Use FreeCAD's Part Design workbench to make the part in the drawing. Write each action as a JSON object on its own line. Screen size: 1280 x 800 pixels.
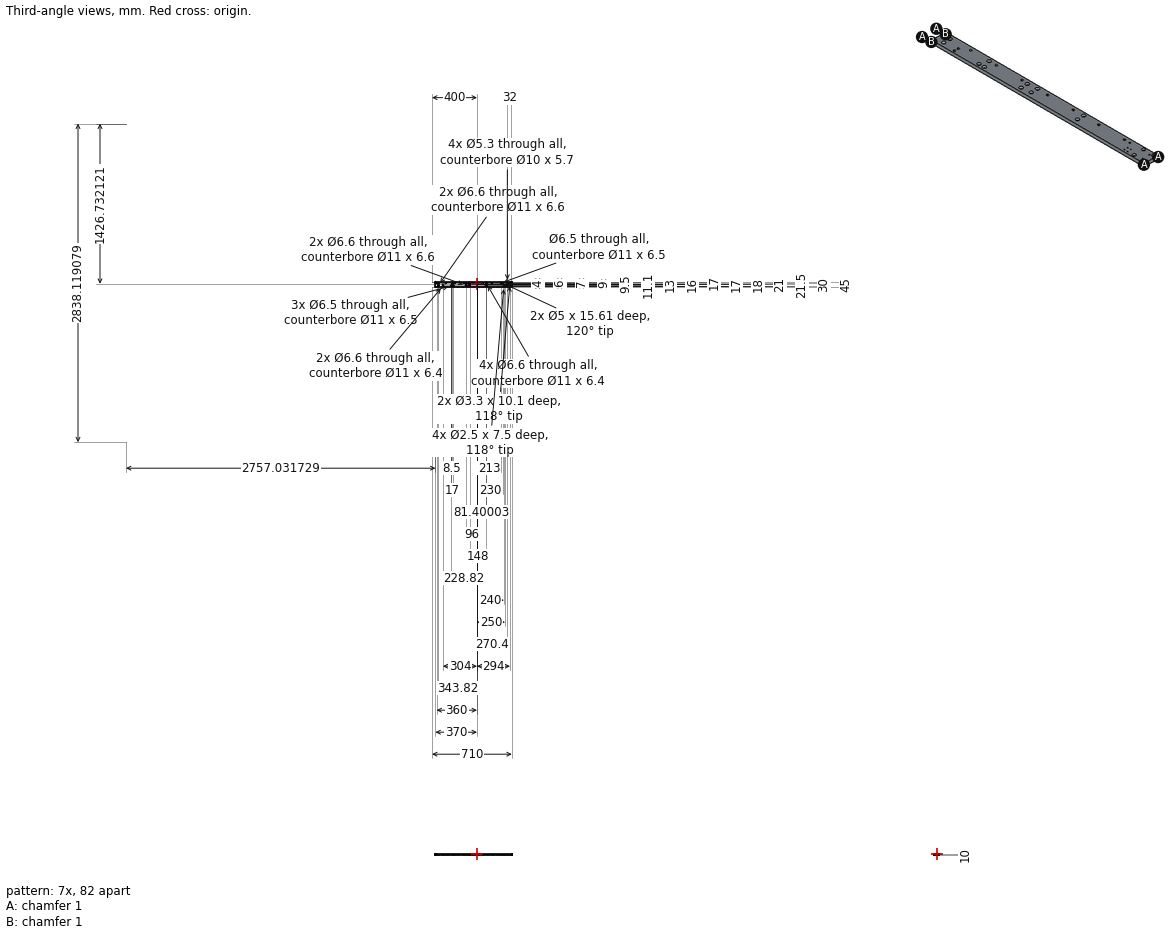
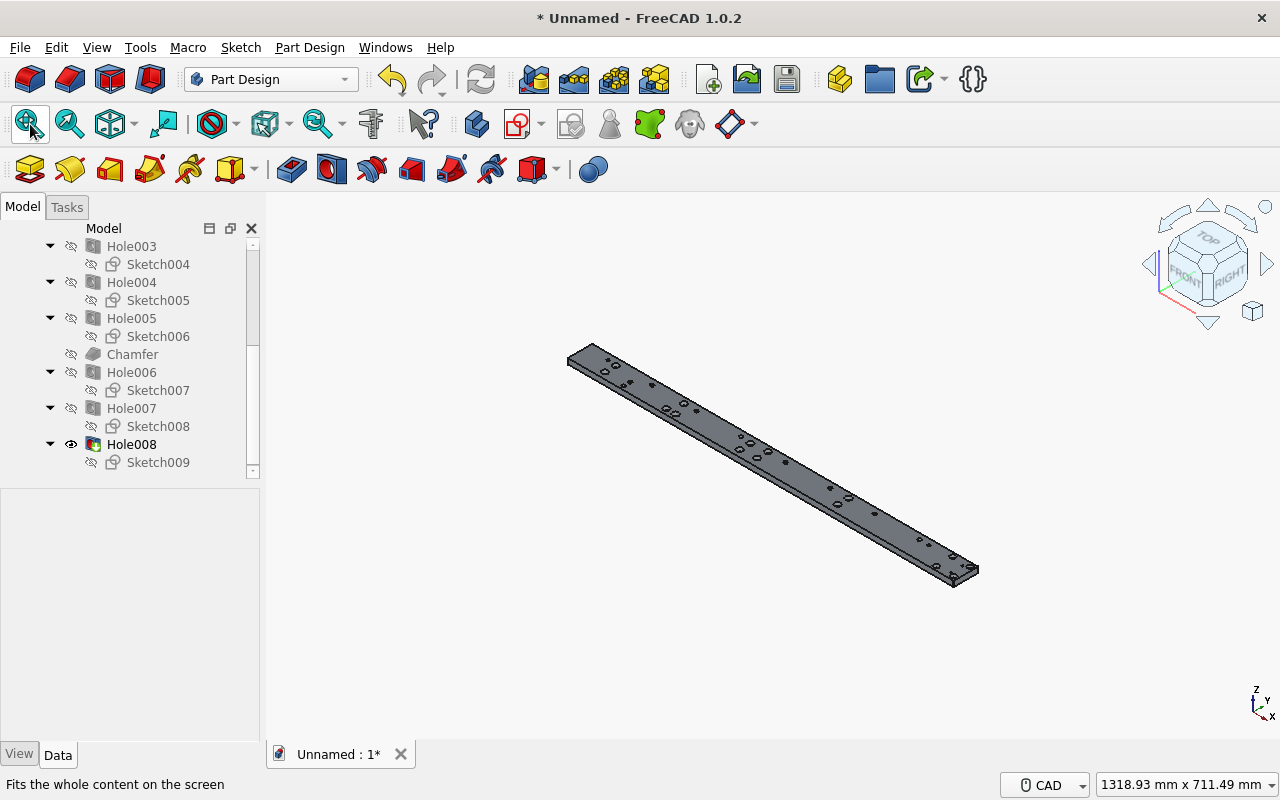
{"action": "left_click", "coordinate": [883, 525]}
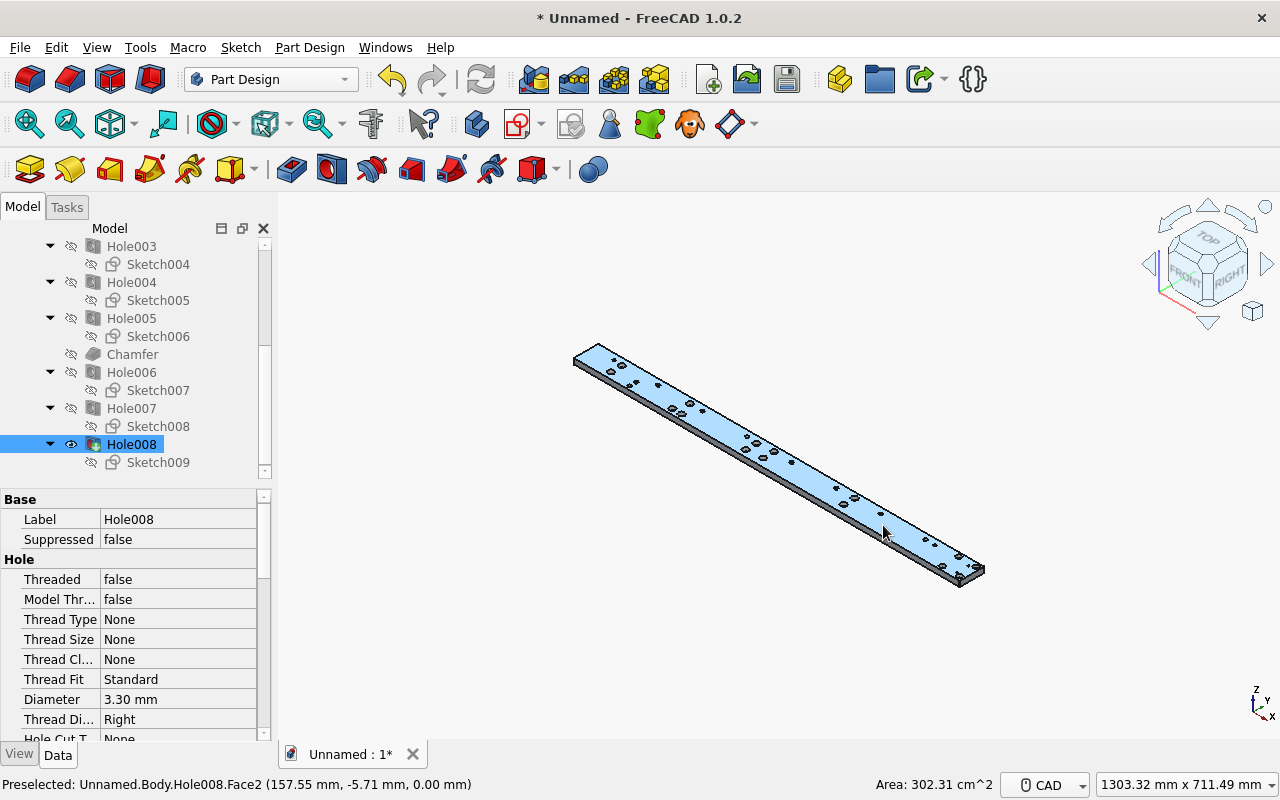
{"action": "left_click", "coordinate": [518, 124]}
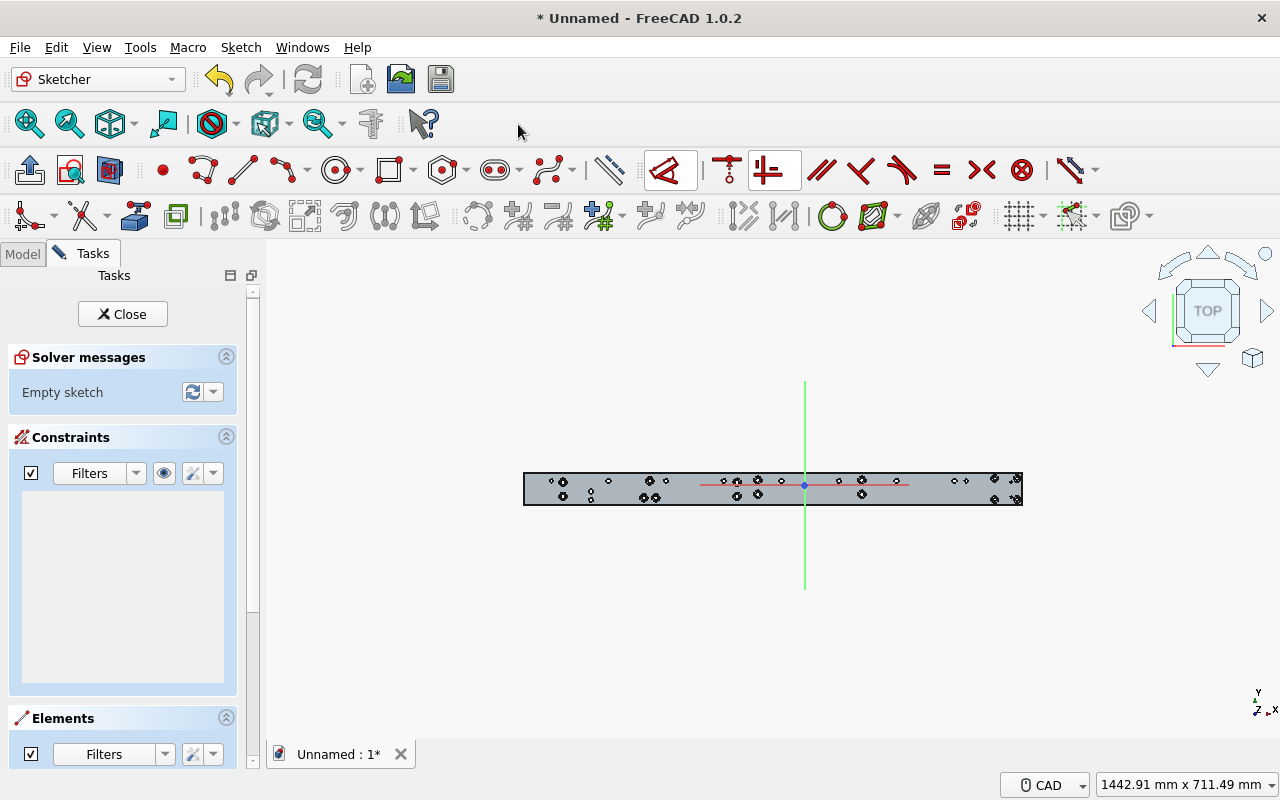
{"action": "scroll", "coordinate": [902, 491], "scroll_direction": "down", "scroll_amount": 9}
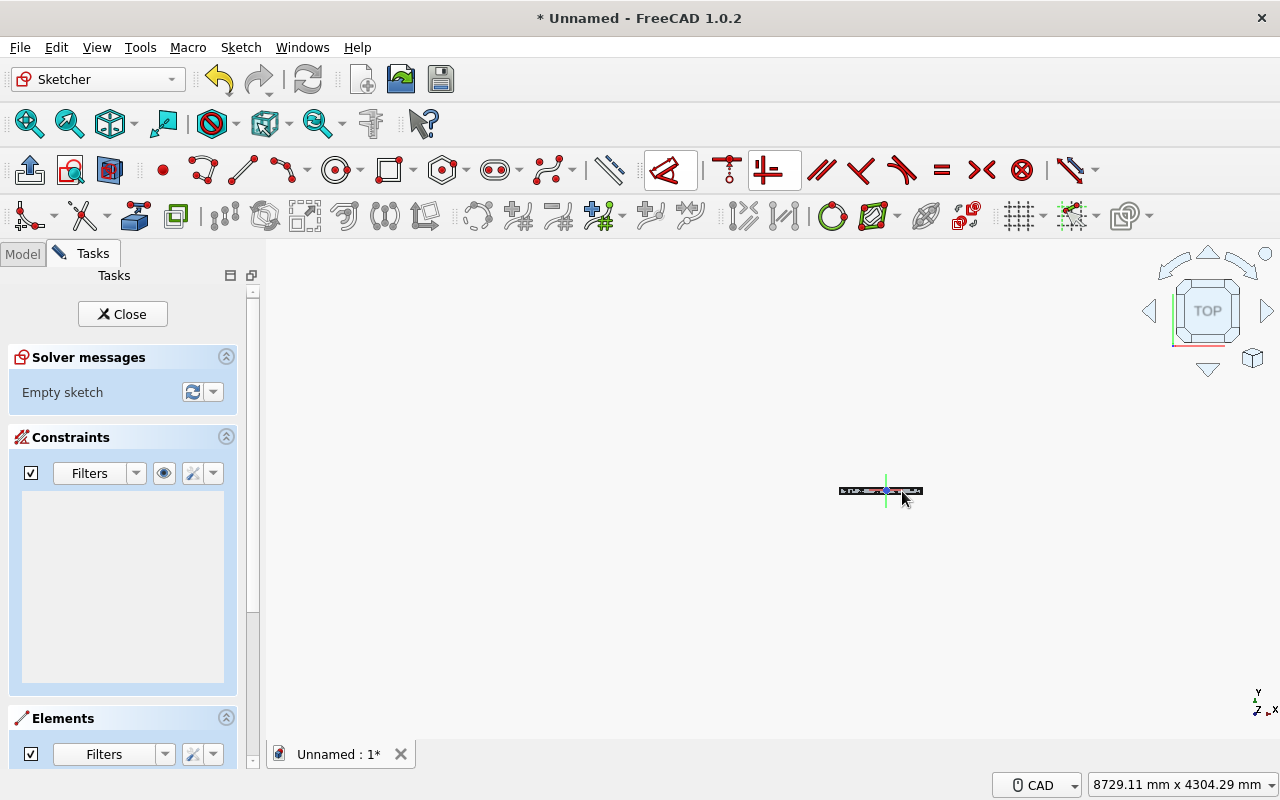
{"action": "left_click", "coordinate": [390, 170]}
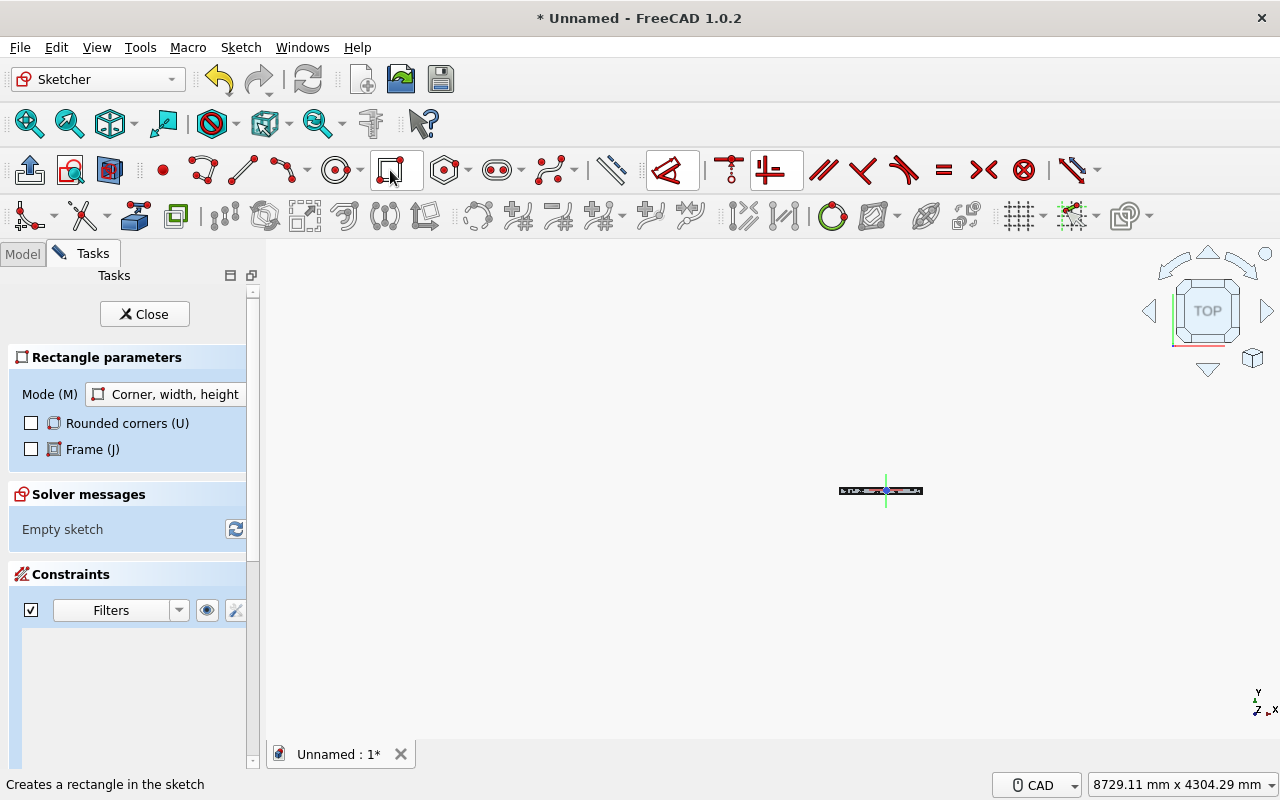
{"action": "left_click", "coordinate": [523, 325]}
{"action": "left_click", "coordinate": [843, 654]}
{"action": "key", "text": "Escape"}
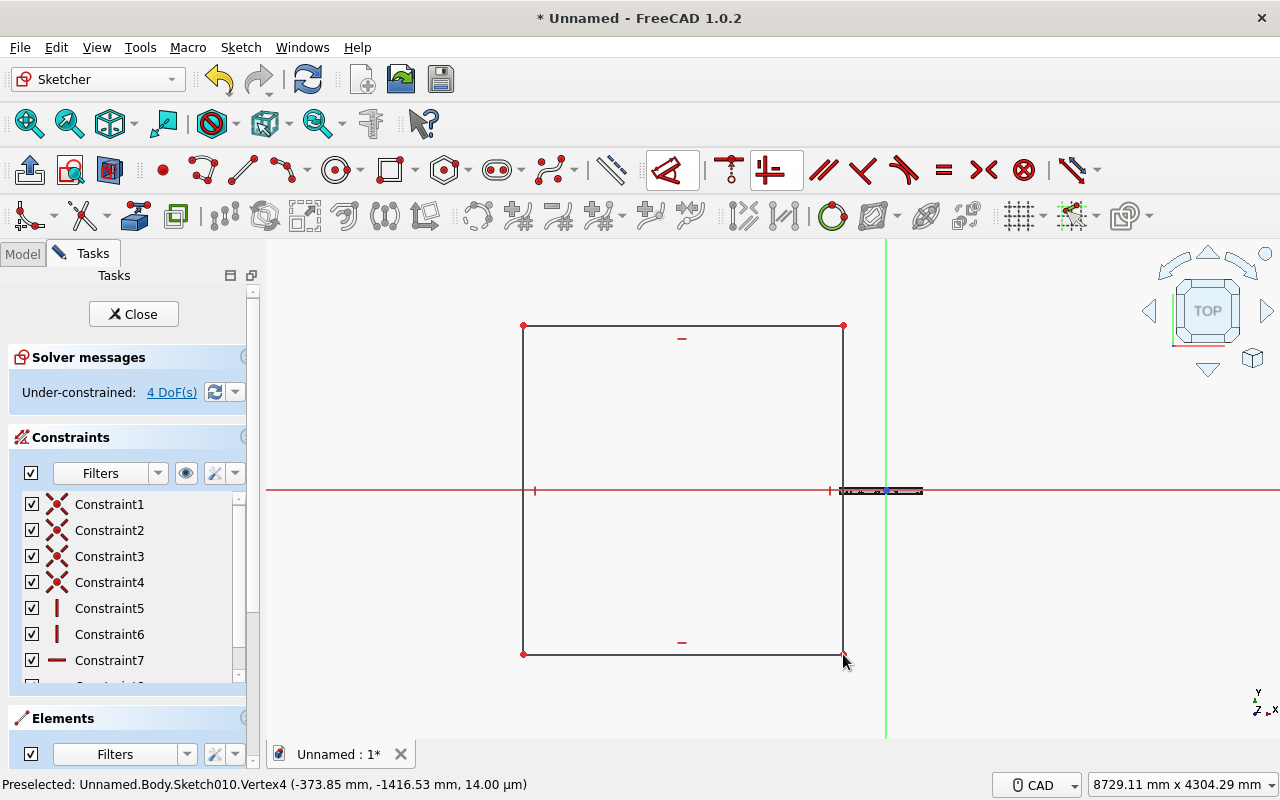
{"action": "left_click", "coordinate": [843, 655]}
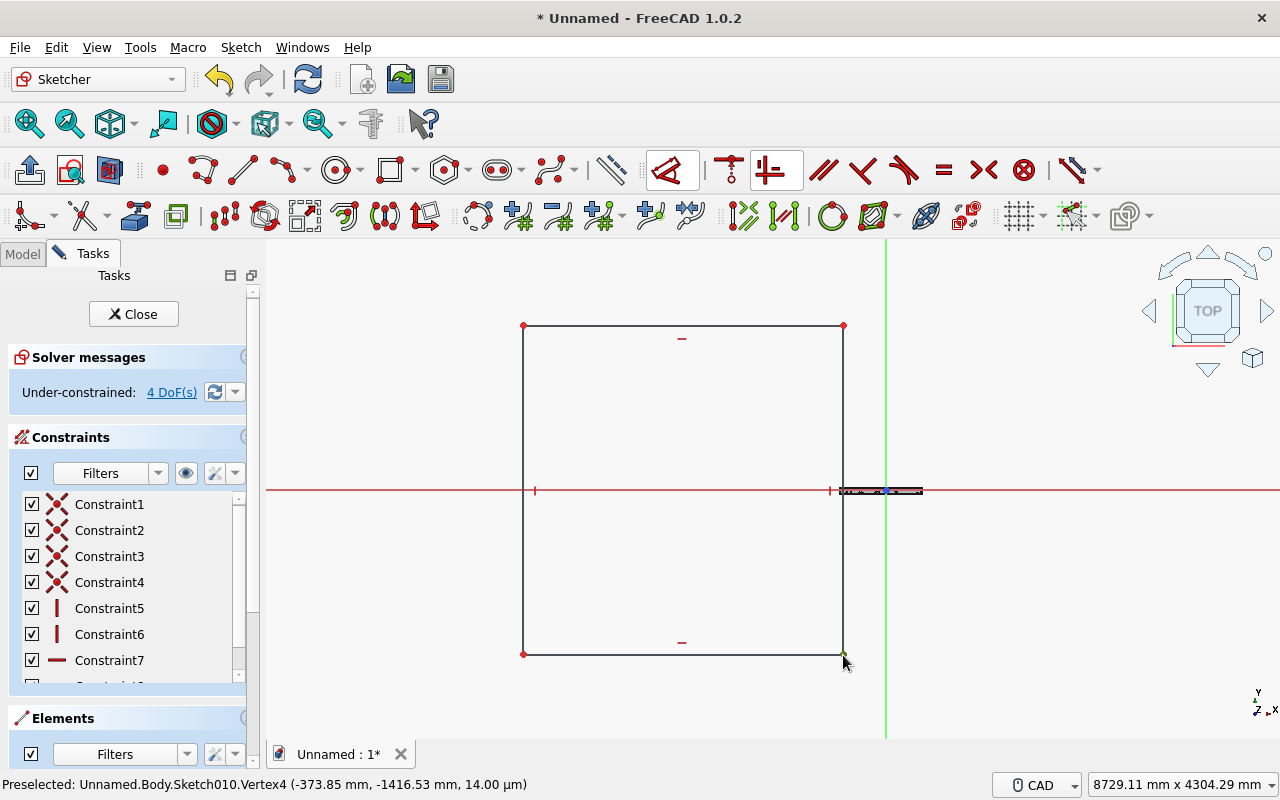
{"action": "left_click", "coordinate": [694, 170]}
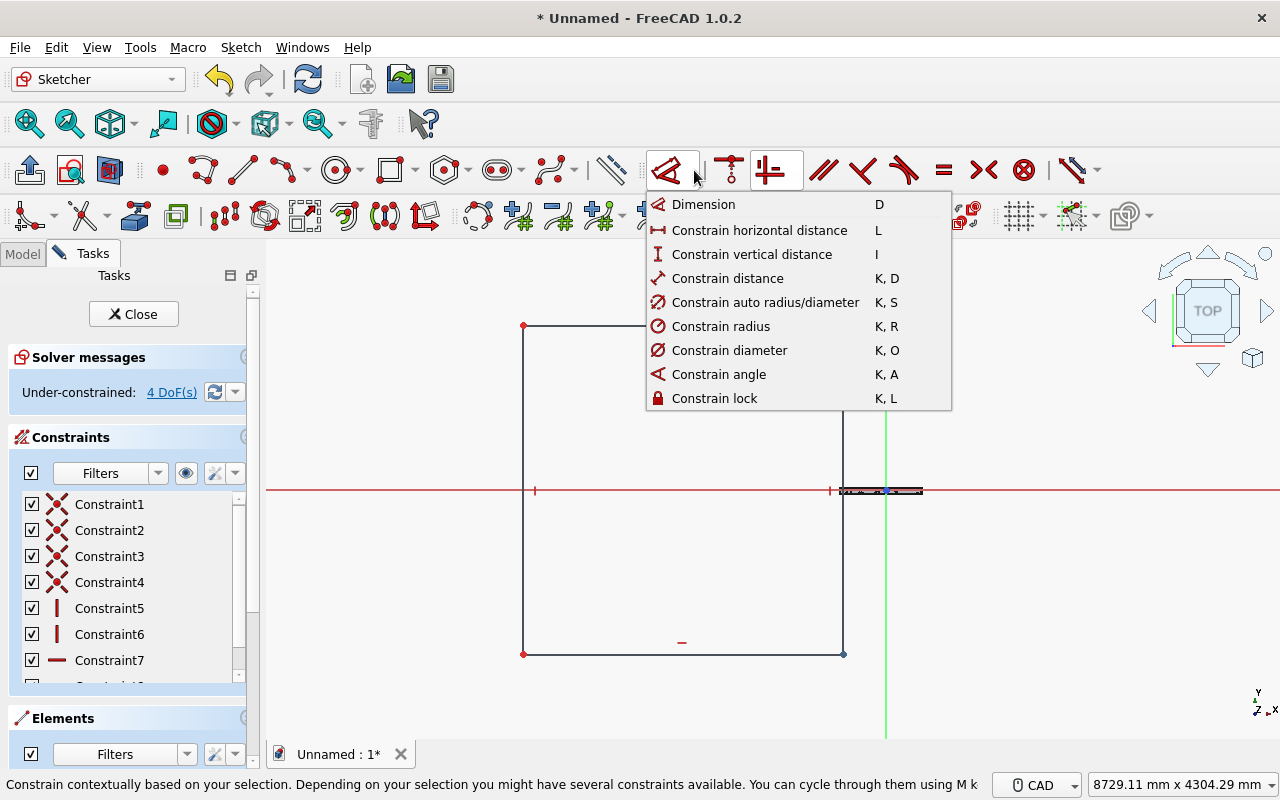
{"action": "left_click", "coordinate": [799, 230]}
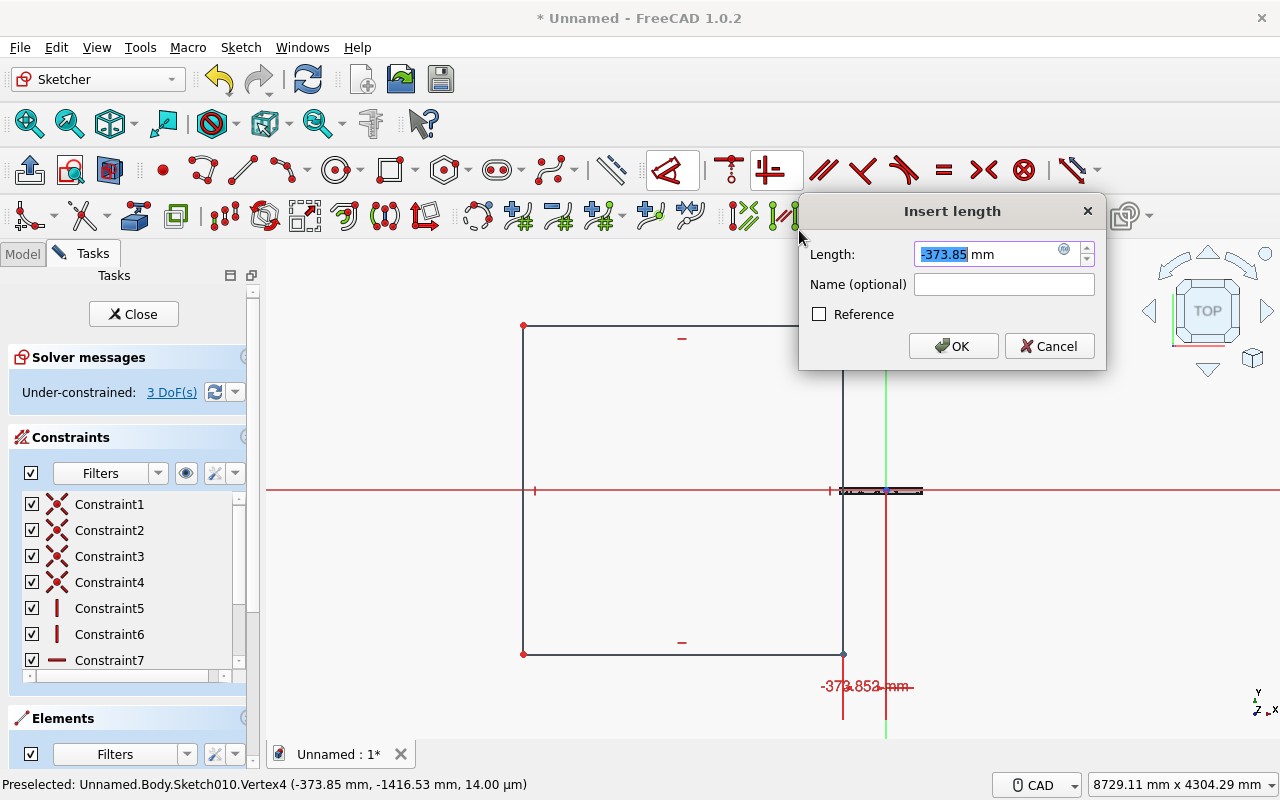
{"action": "type", "text": "-370"}
{"action": "key", "text": "Return"}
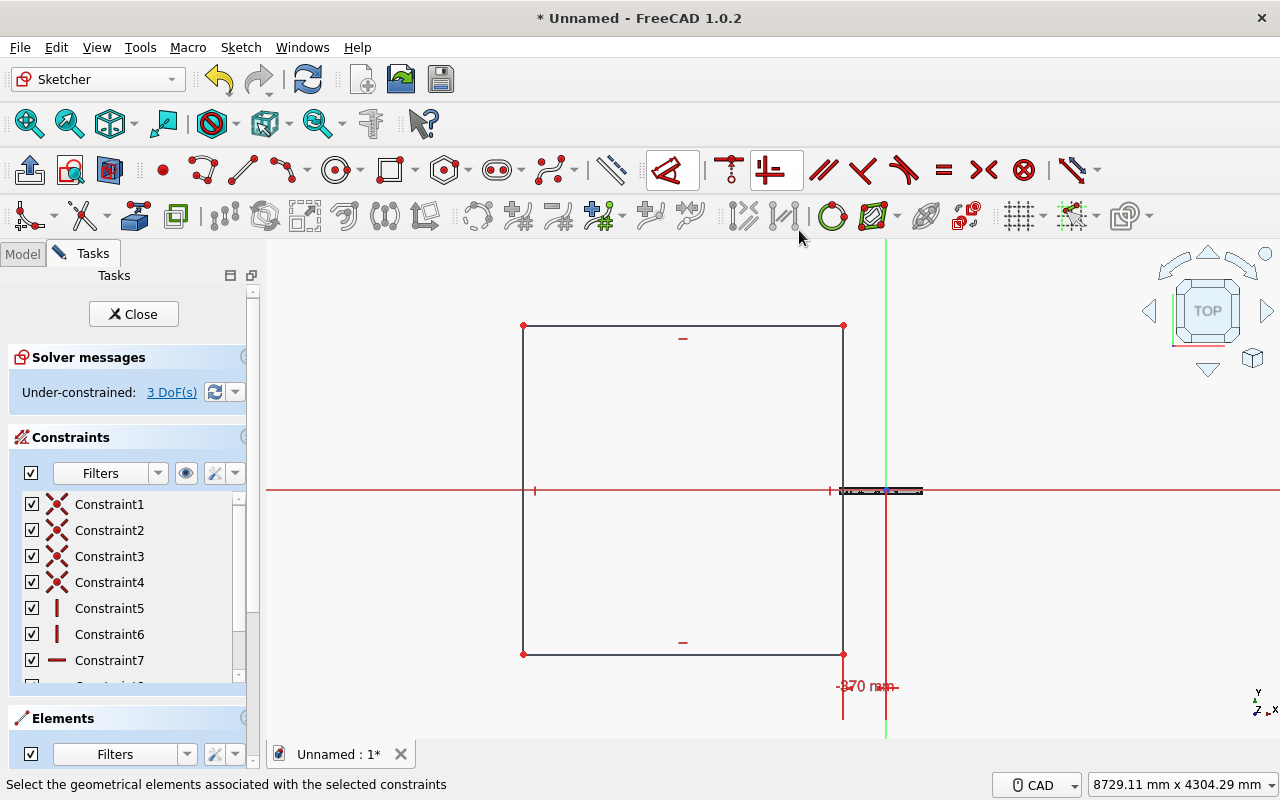
{"action": "left_click", "coordinate": [523, 425]}